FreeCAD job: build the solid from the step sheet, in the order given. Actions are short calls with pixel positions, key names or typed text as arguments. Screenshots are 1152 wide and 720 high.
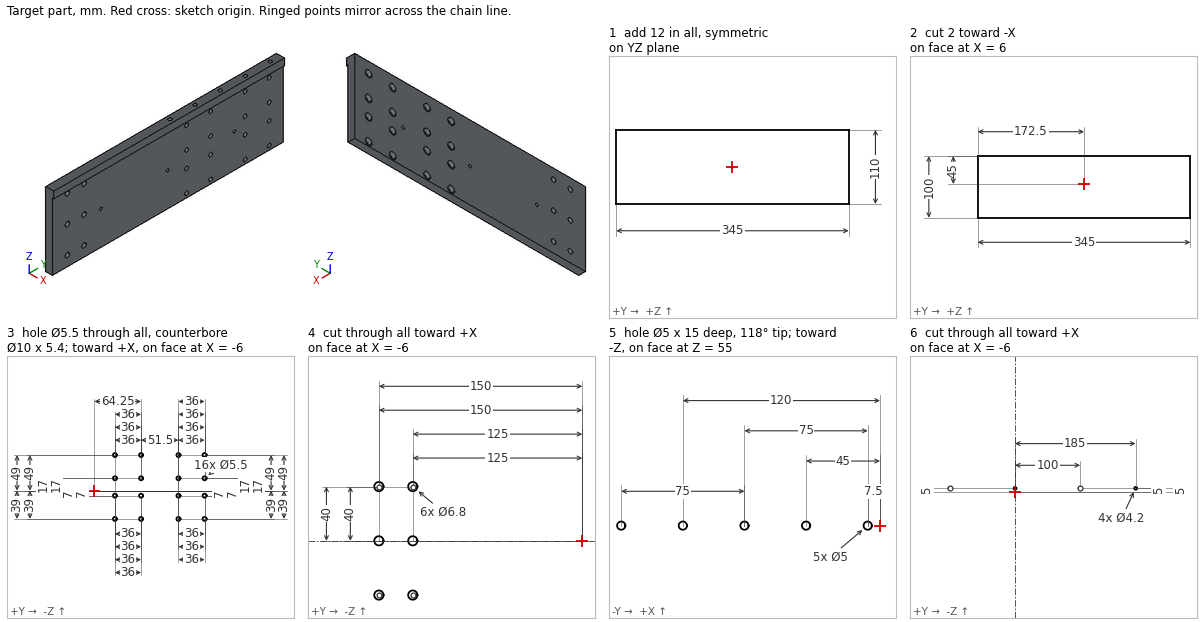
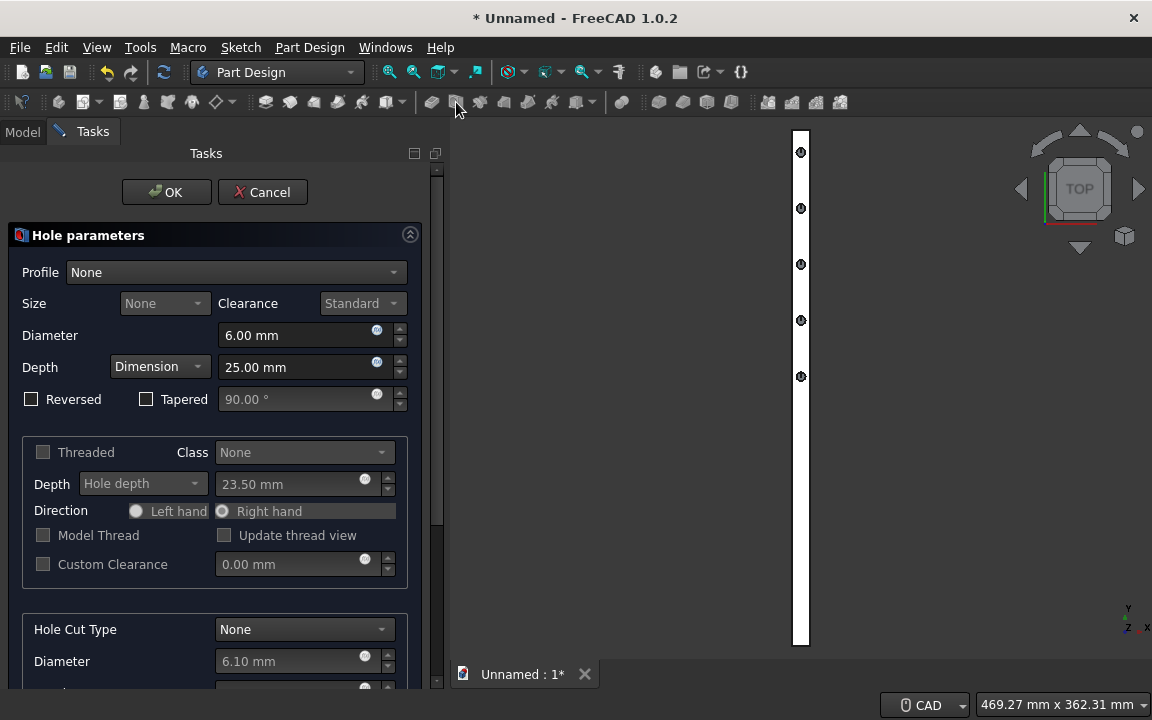
triple_click(305, 335)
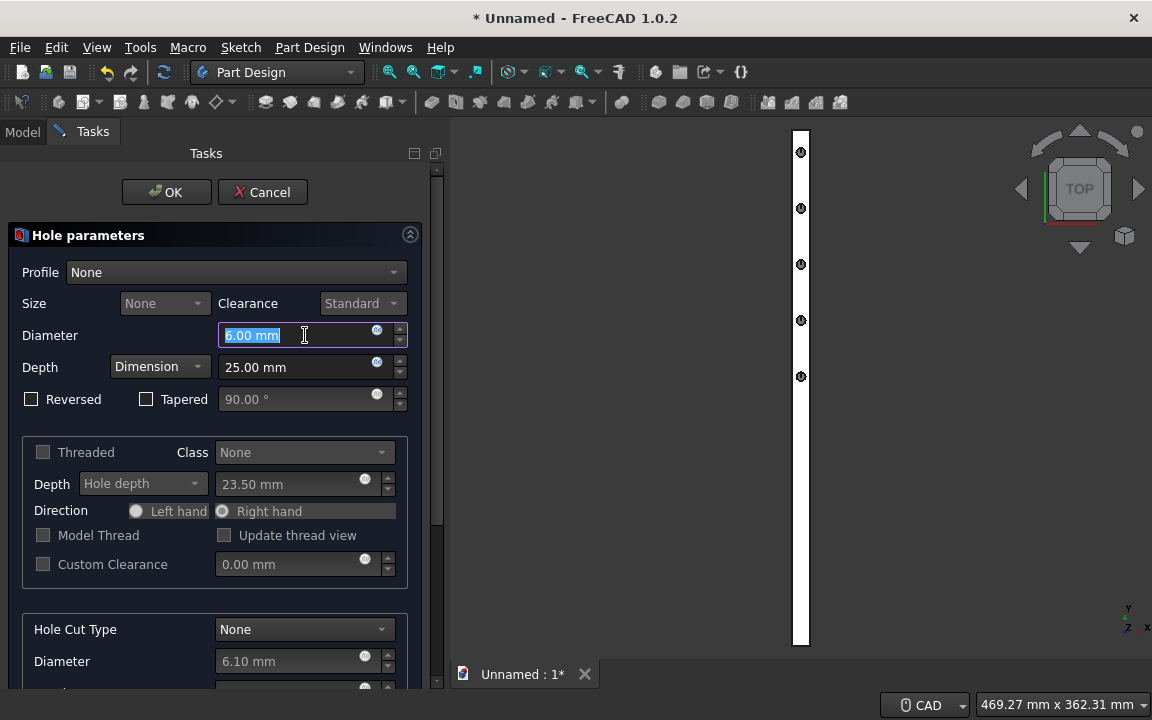
text(5)
key(Tab)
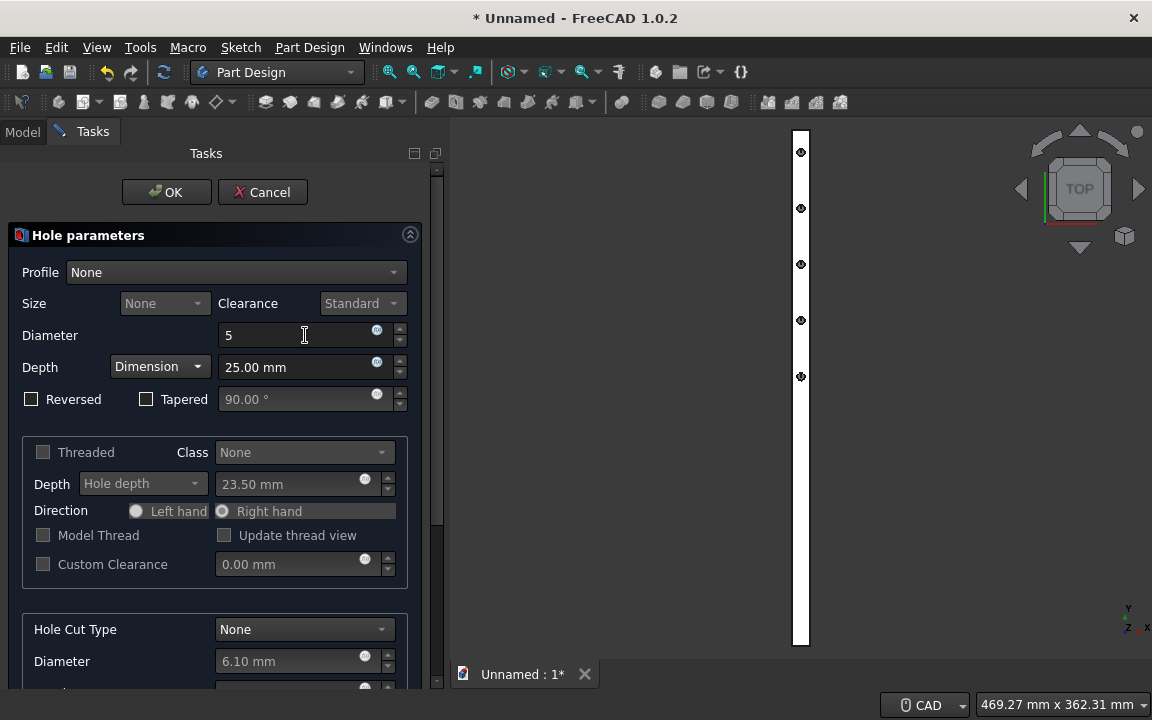
triple_click(305, 367)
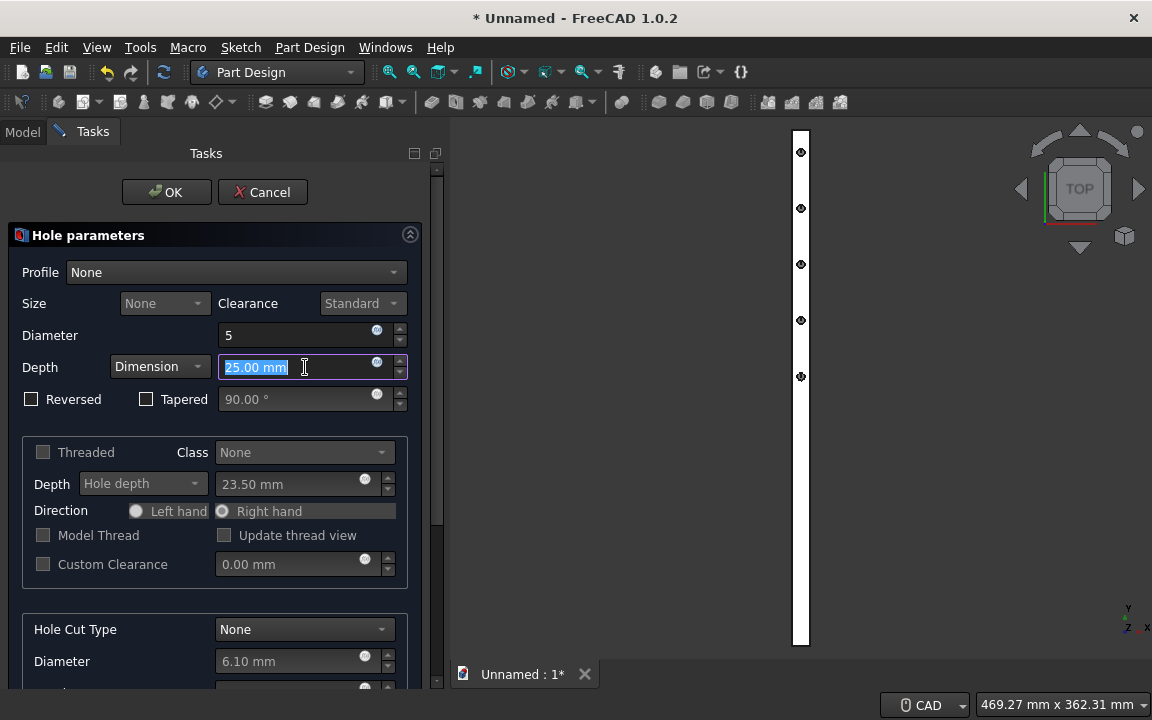
text(15)
key(Tab)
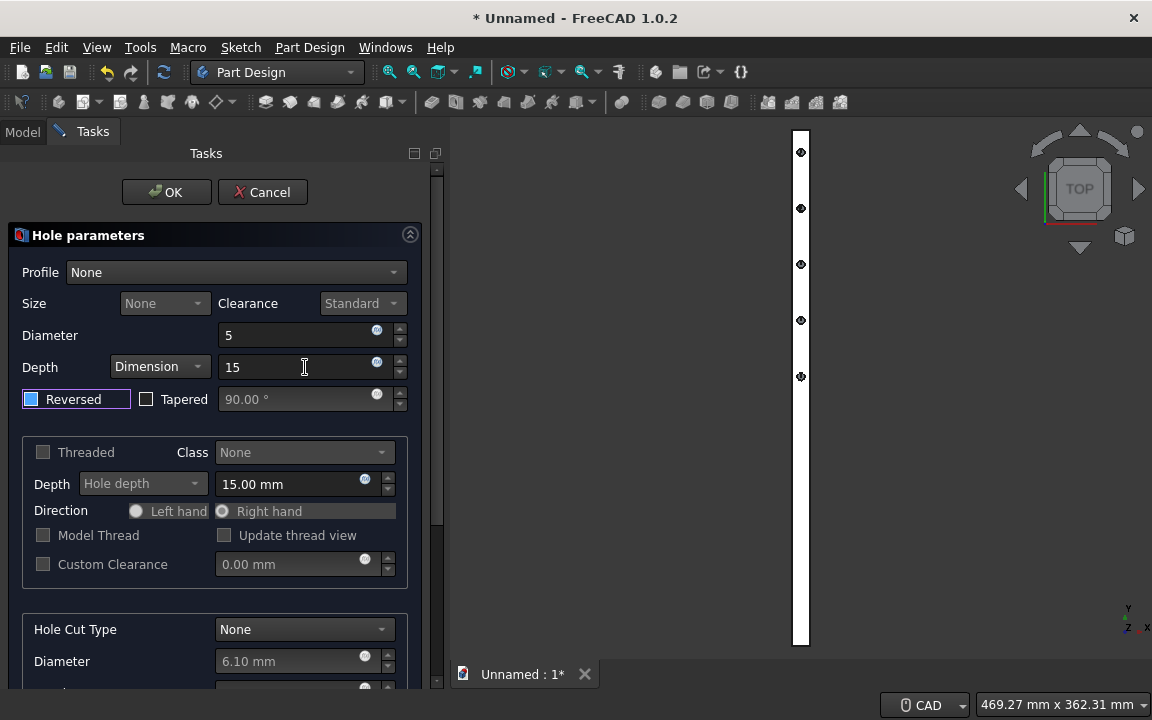
click(167, 192)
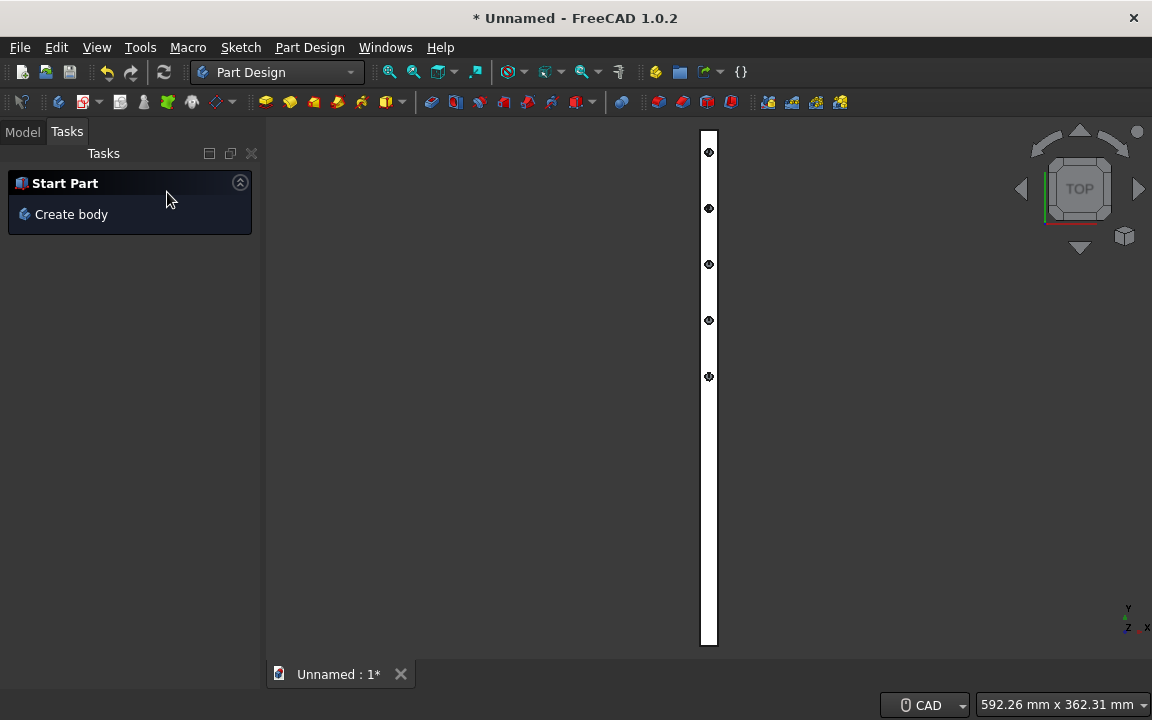
key(6)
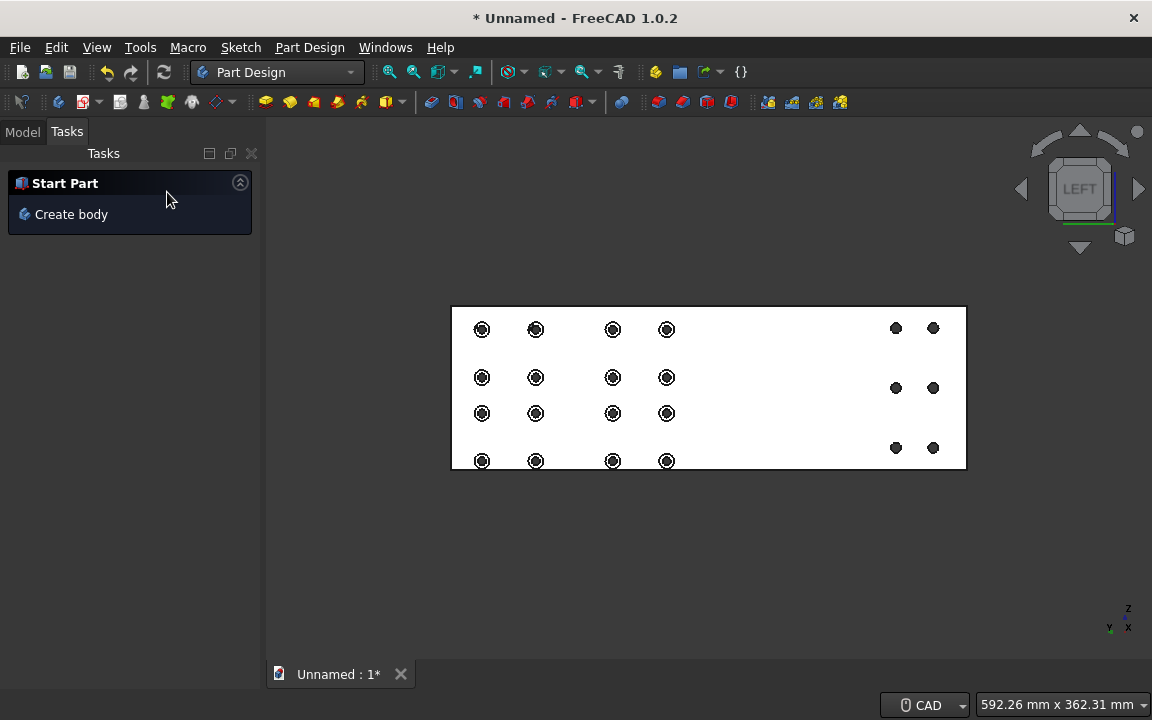
click(783, 387)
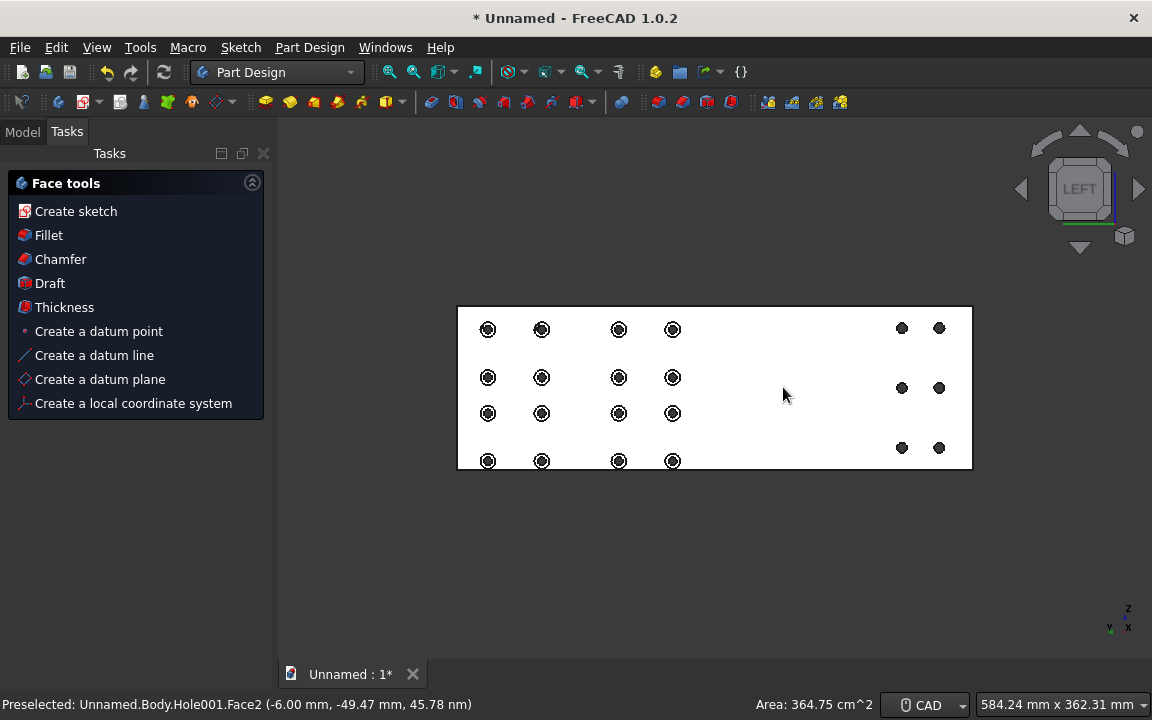
click(84, 102)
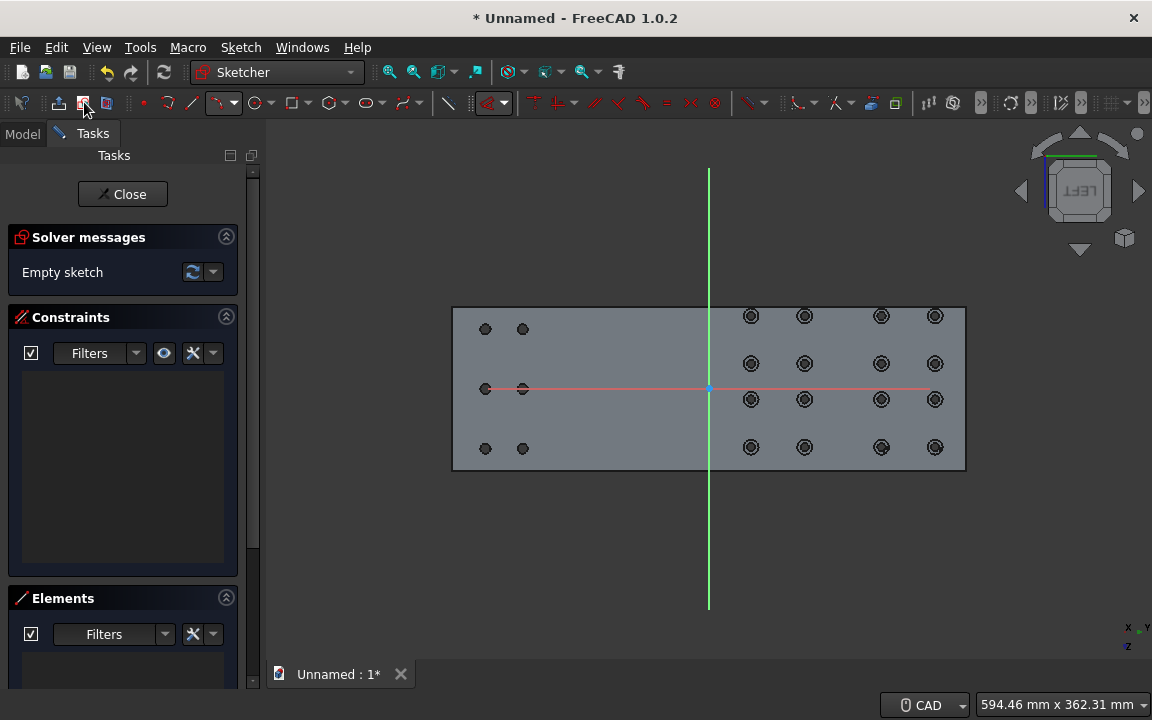
scroll(294, 413, down, 1)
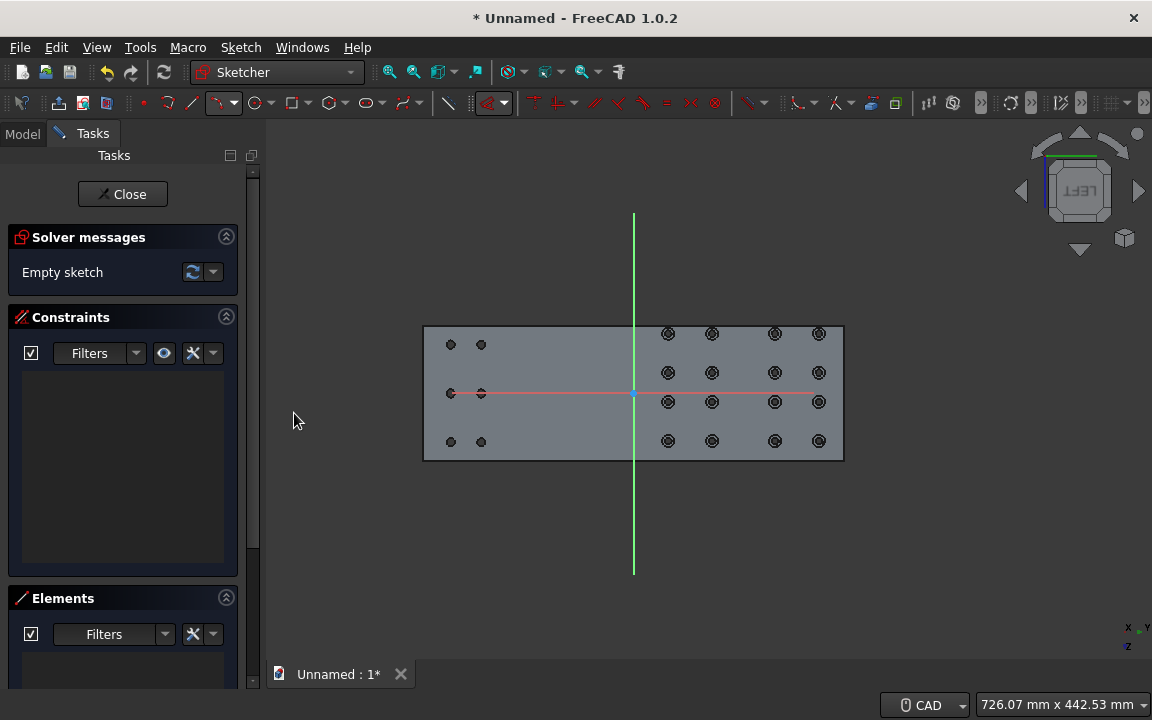
scroll(777, 389, up, 2)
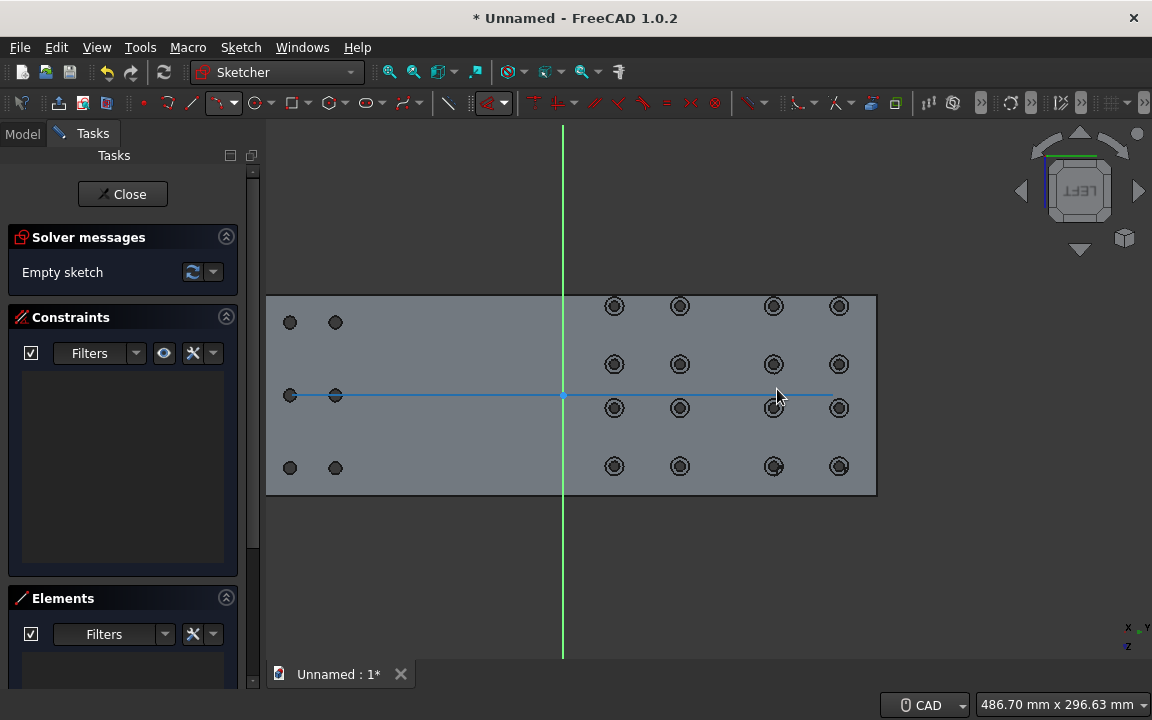
click(256, 104)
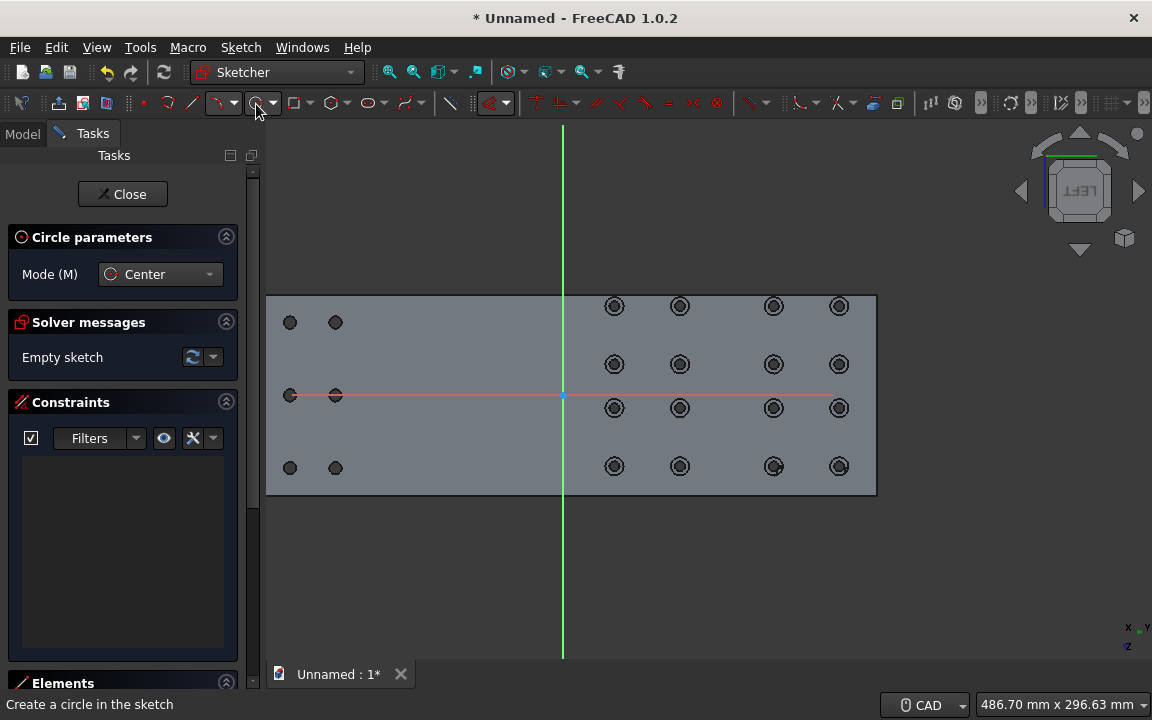
scroll(900, 386, up, 9)